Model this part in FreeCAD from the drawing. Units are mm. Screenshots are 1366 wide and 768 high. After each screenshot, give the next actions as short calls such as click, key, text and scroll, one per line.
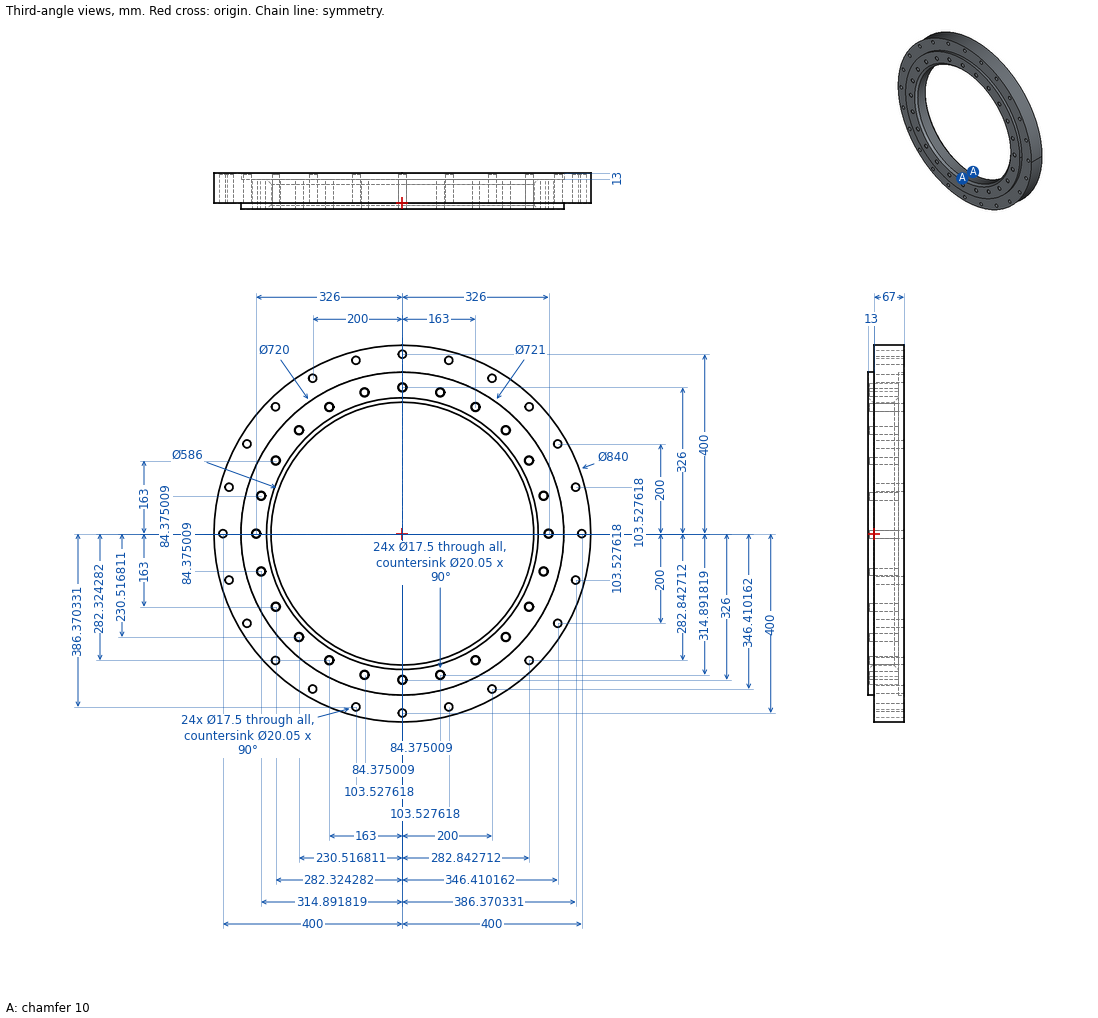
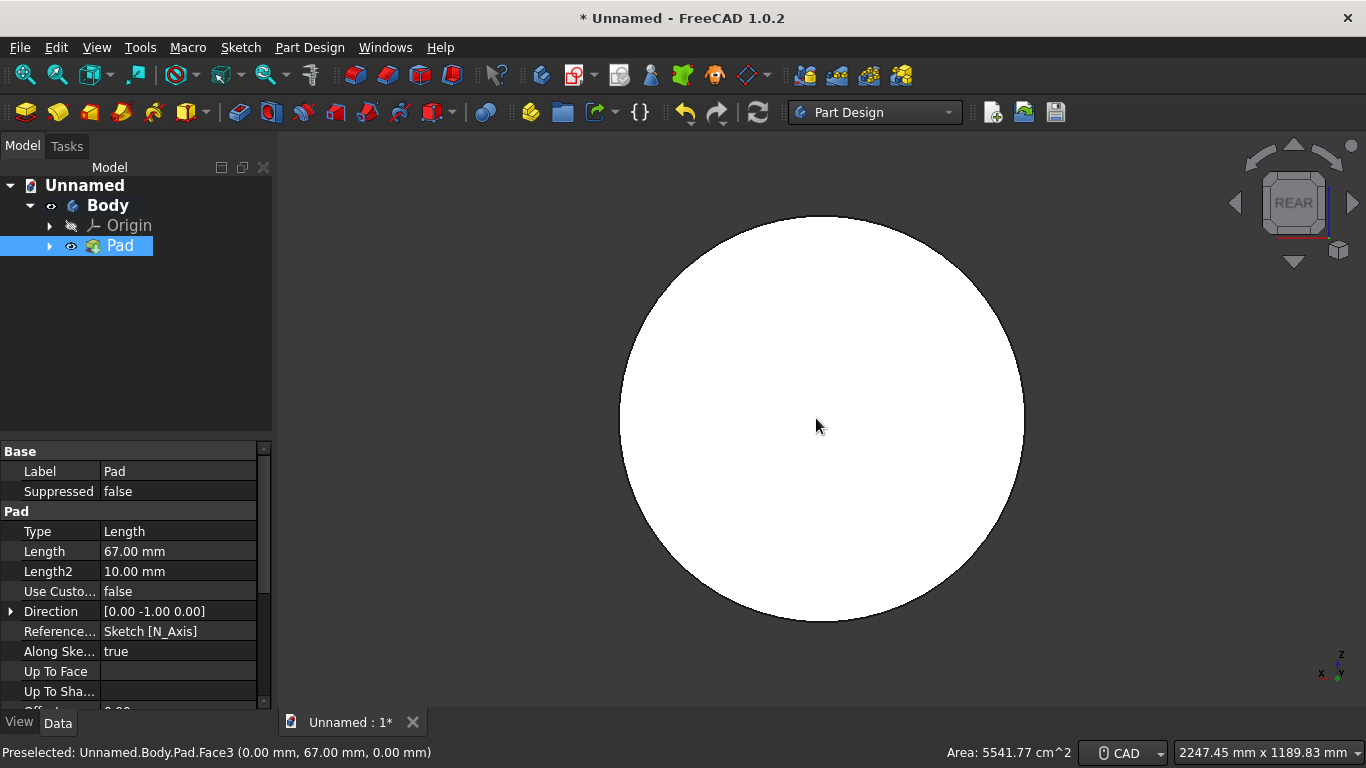
click(574, 76)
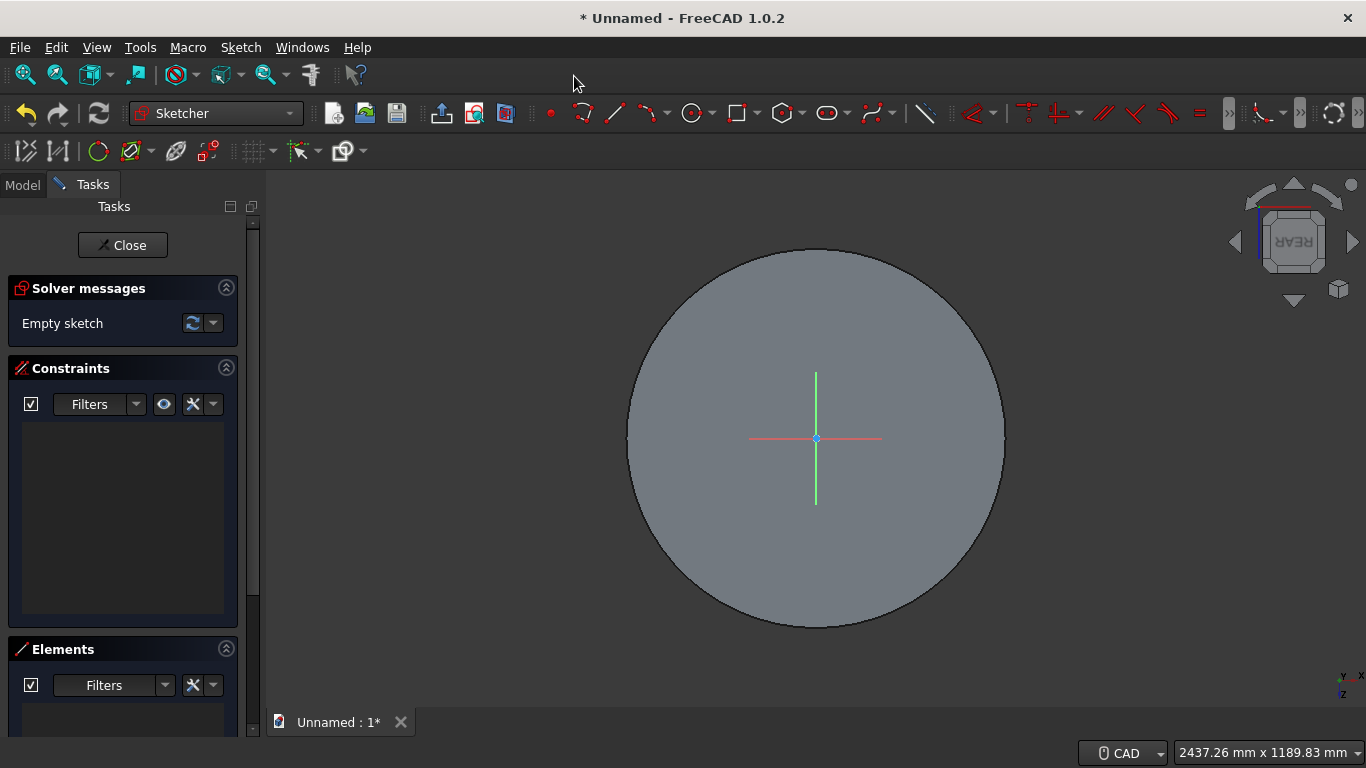
key(g)
key(c)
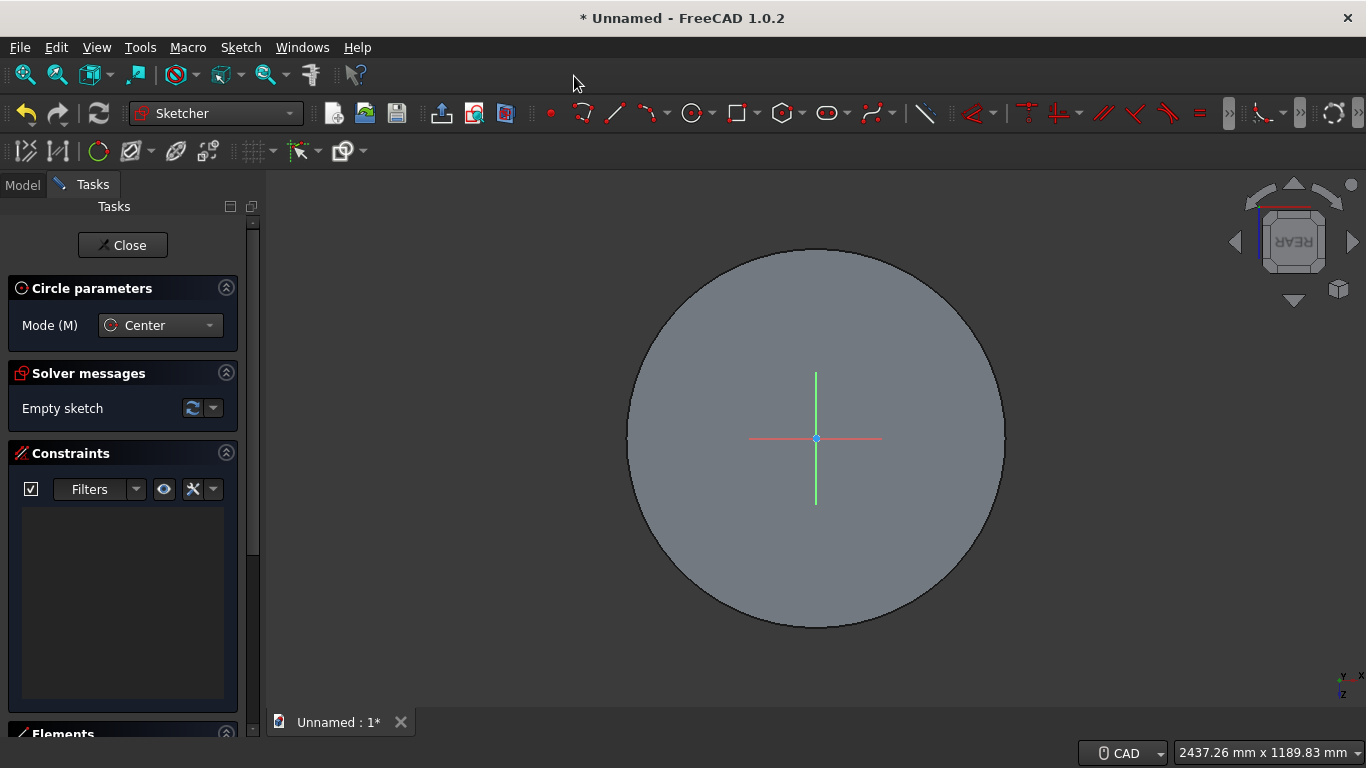
click(816, 439)
click(931, 323)
key(Escape)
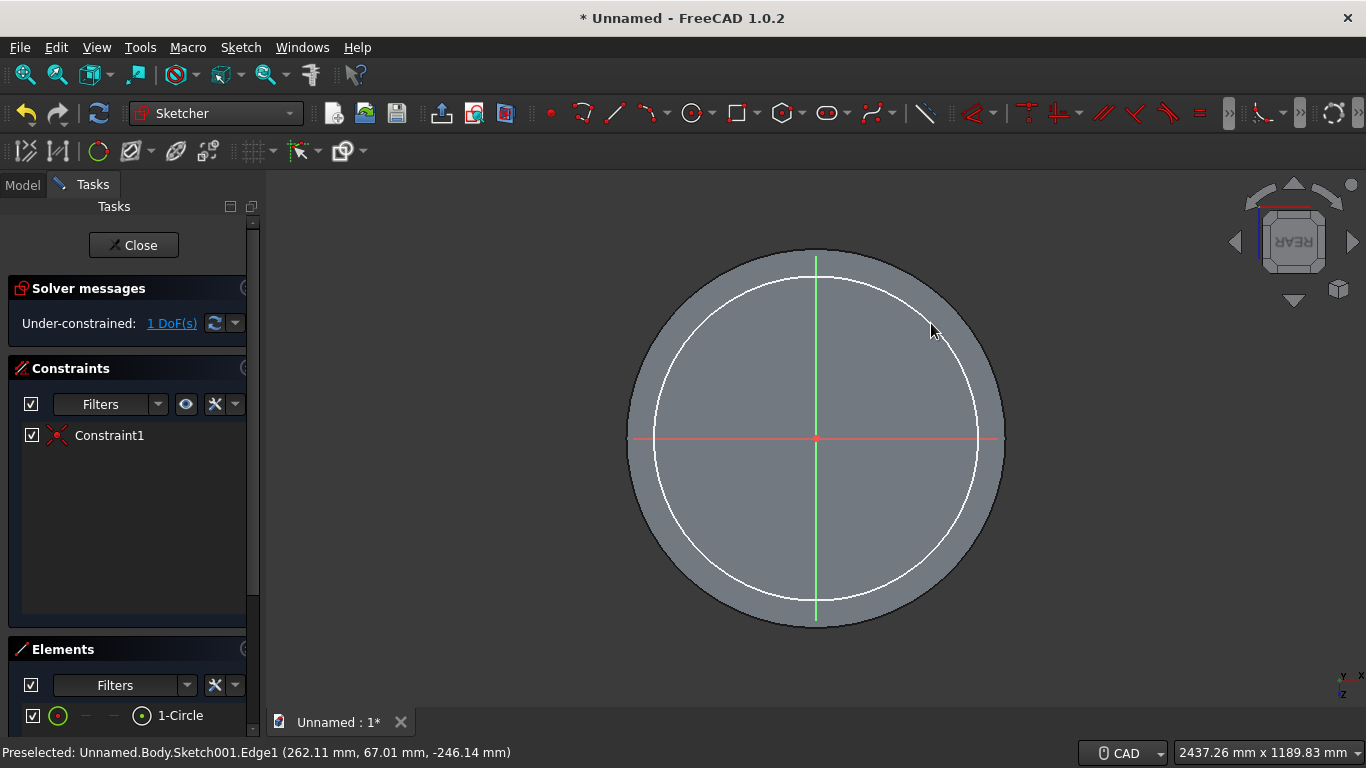
click(930, 323)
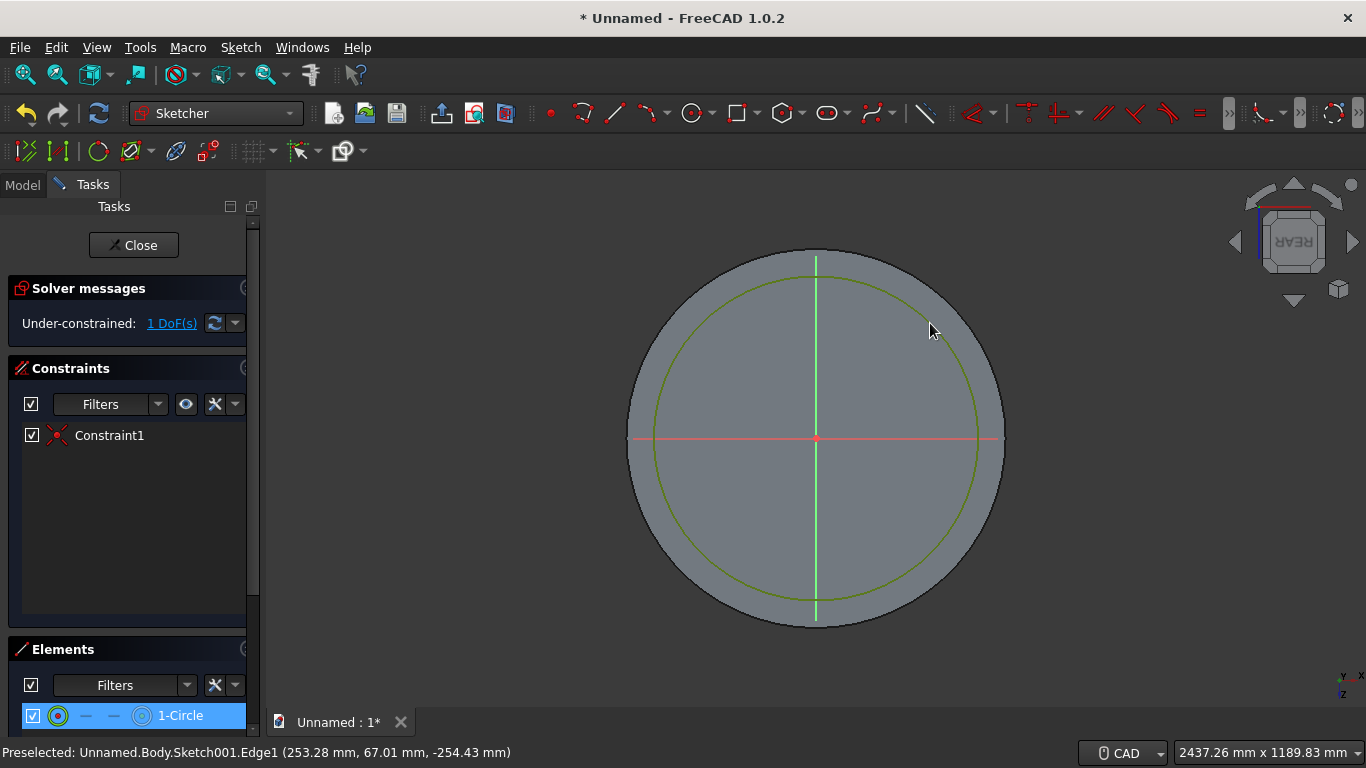
click(996, 114)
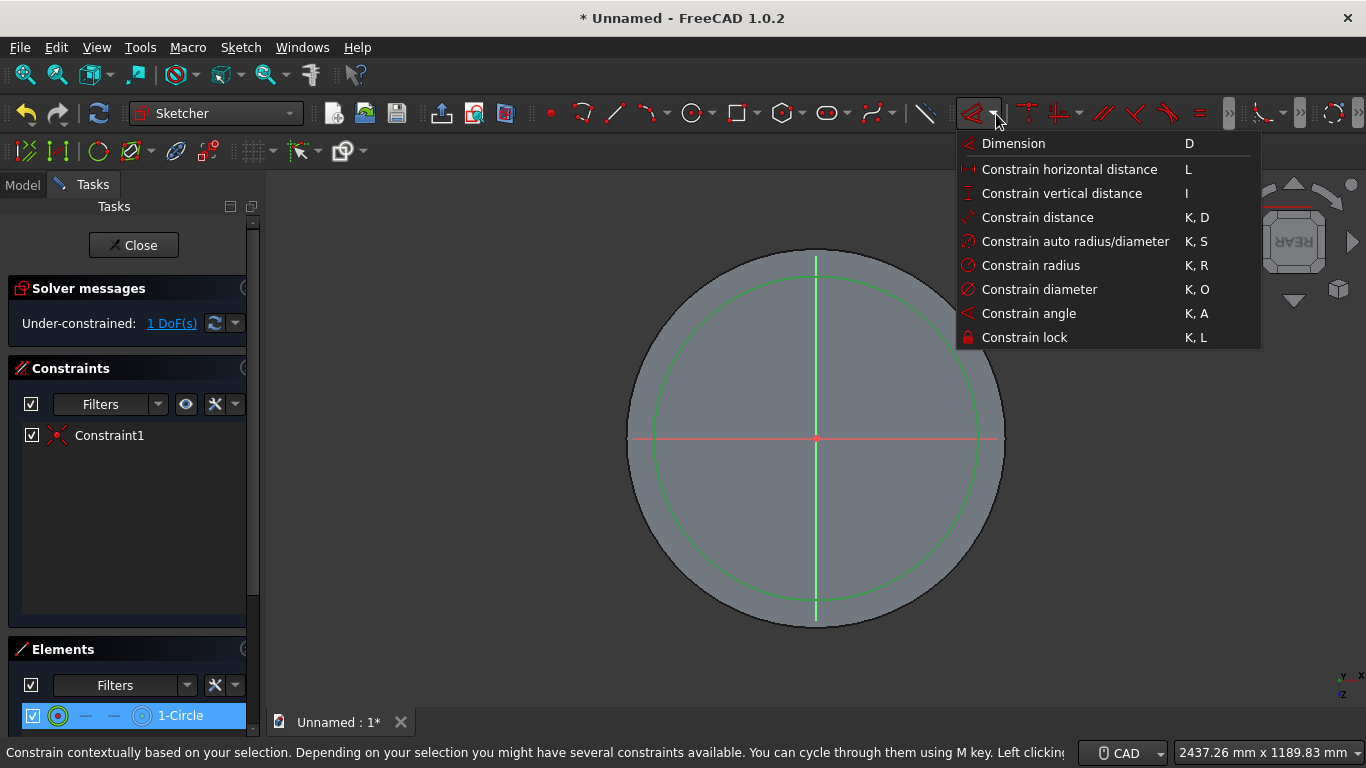
click(1109, 289)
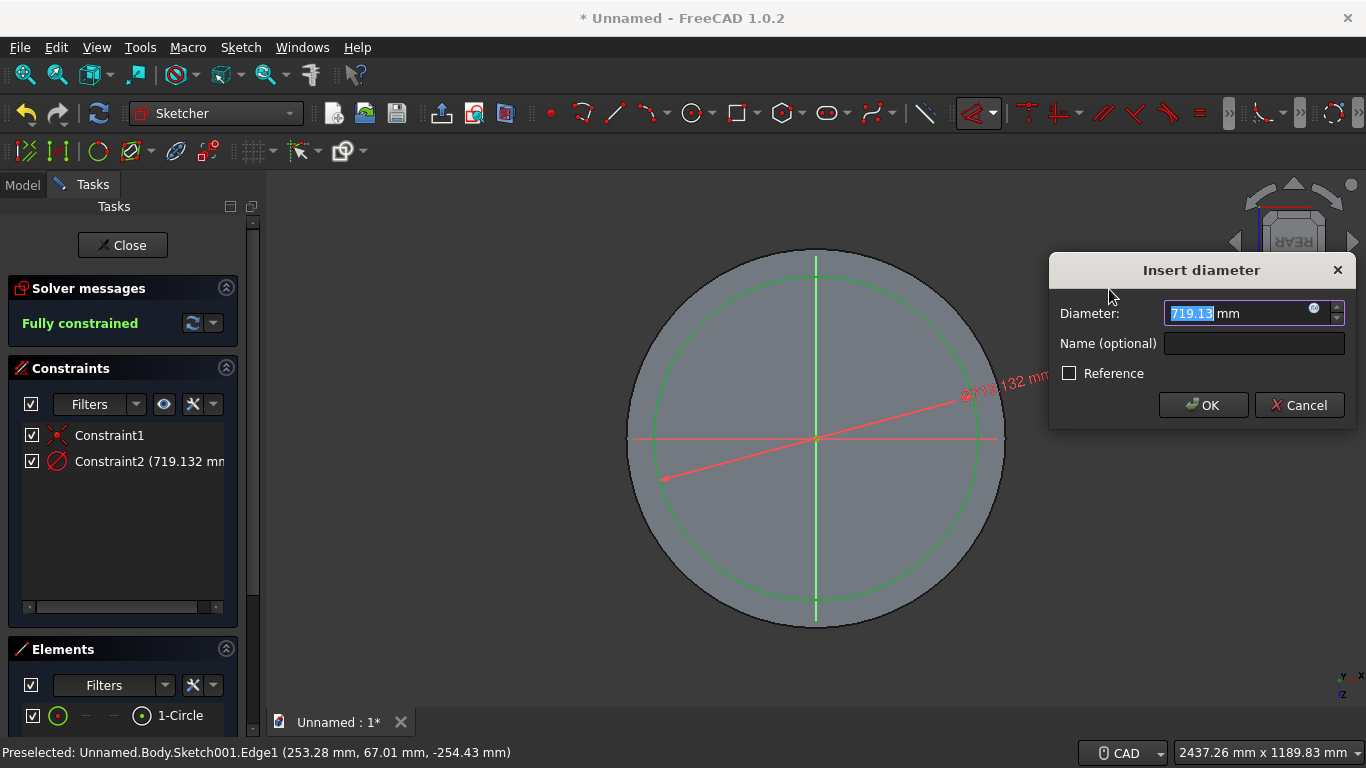
text(721)
key(Return)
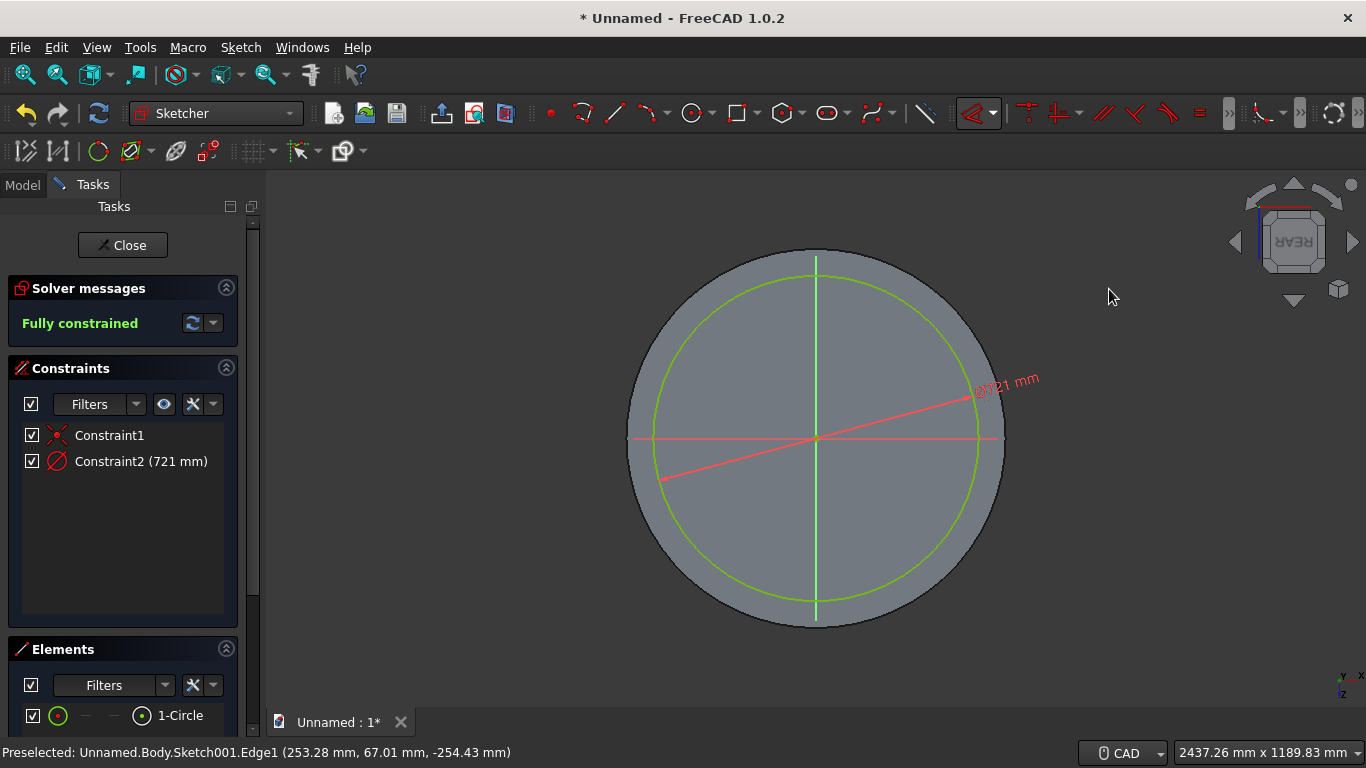
click(123, 245)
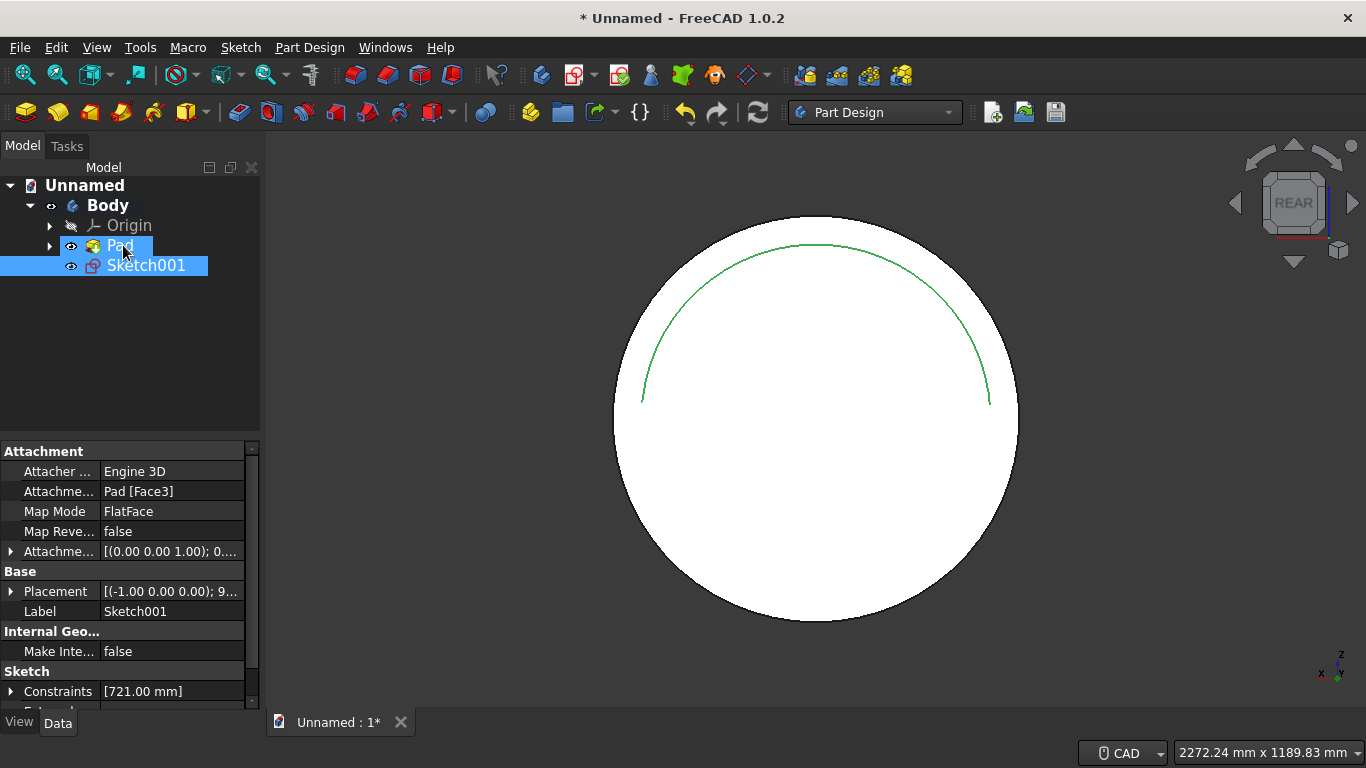
click(240, 112)